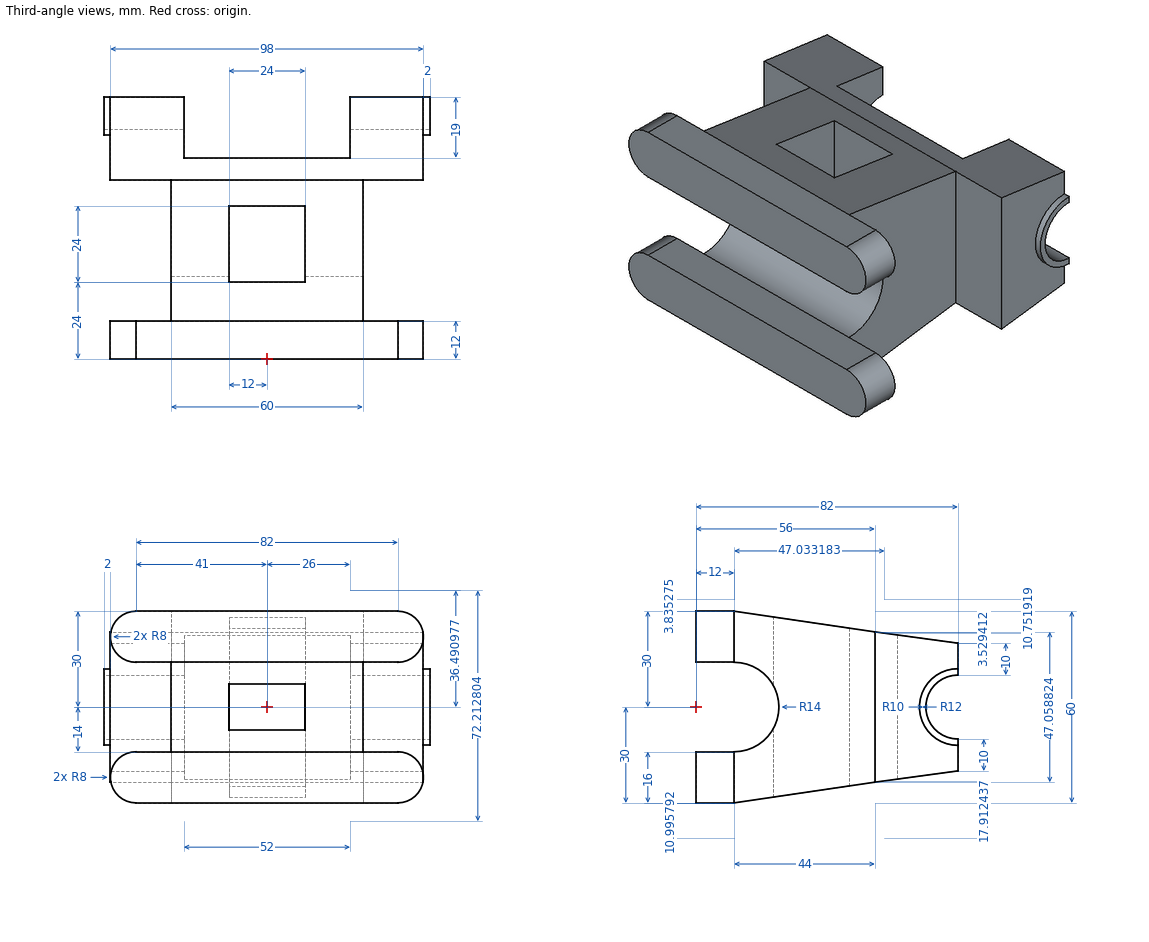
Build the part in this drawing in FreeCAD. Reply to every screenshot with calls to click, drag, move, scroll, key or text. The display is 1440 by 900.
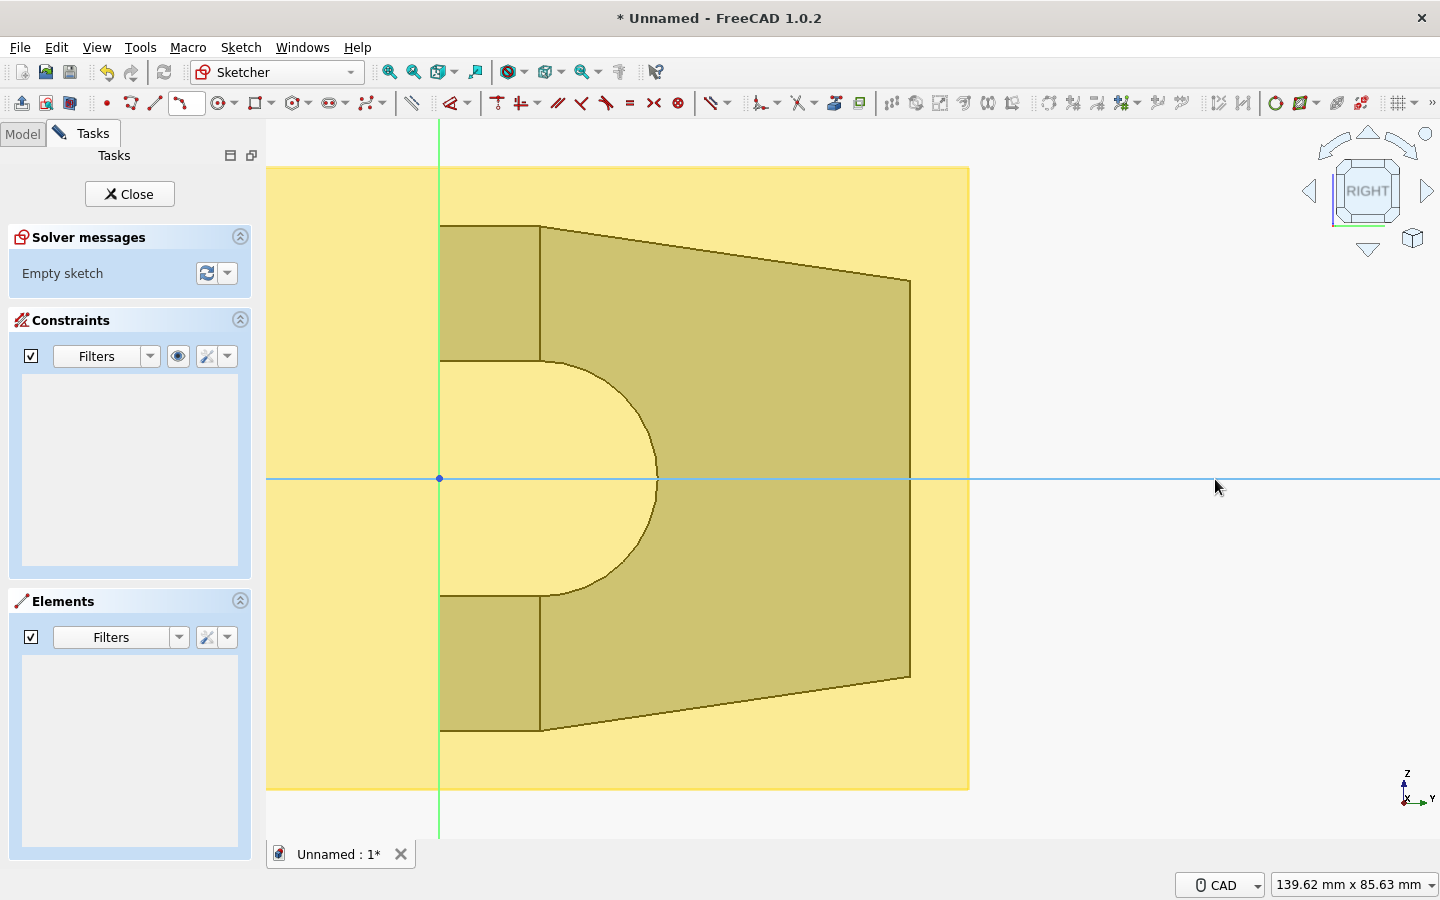
click(132, 104)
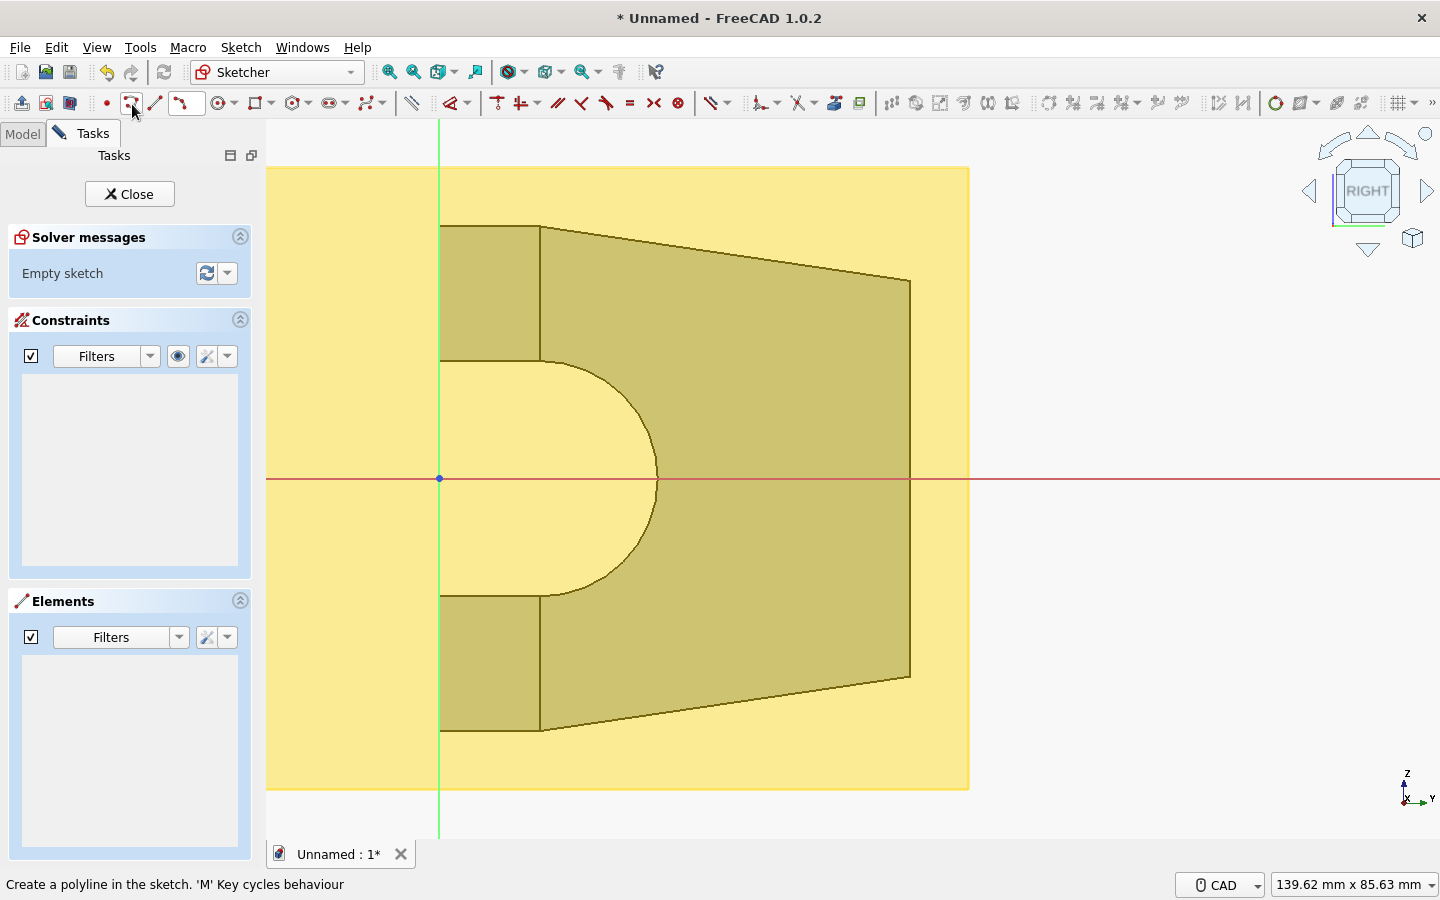
click(1129, 395)
click(1129, 311)
click(910, 281)
click(910, 677)
click(1129, 647)
click(1129, 563)
right_click(1129, 563)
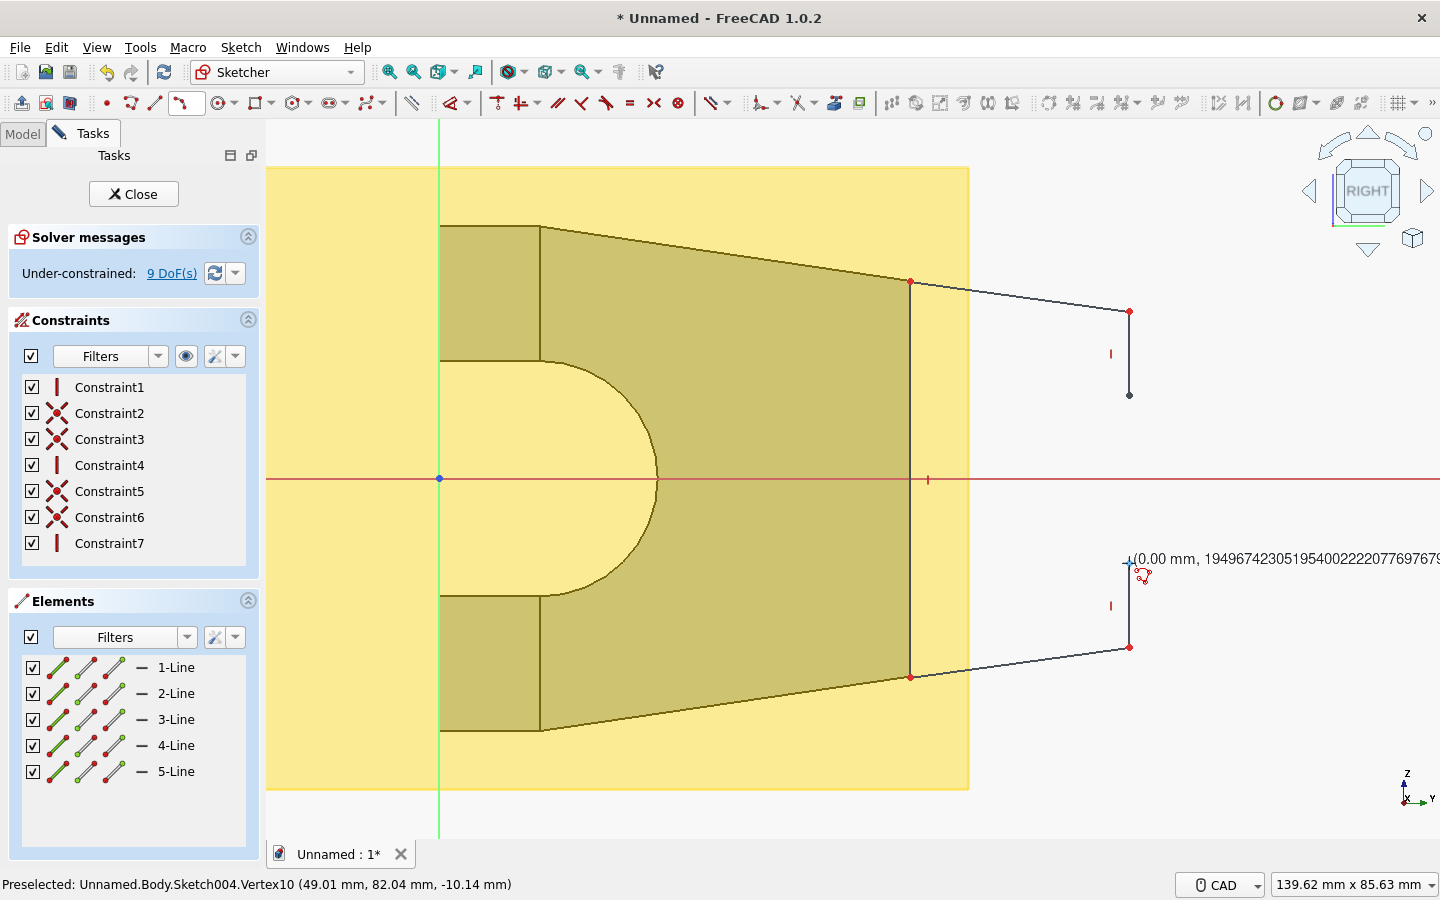
click(180, 104)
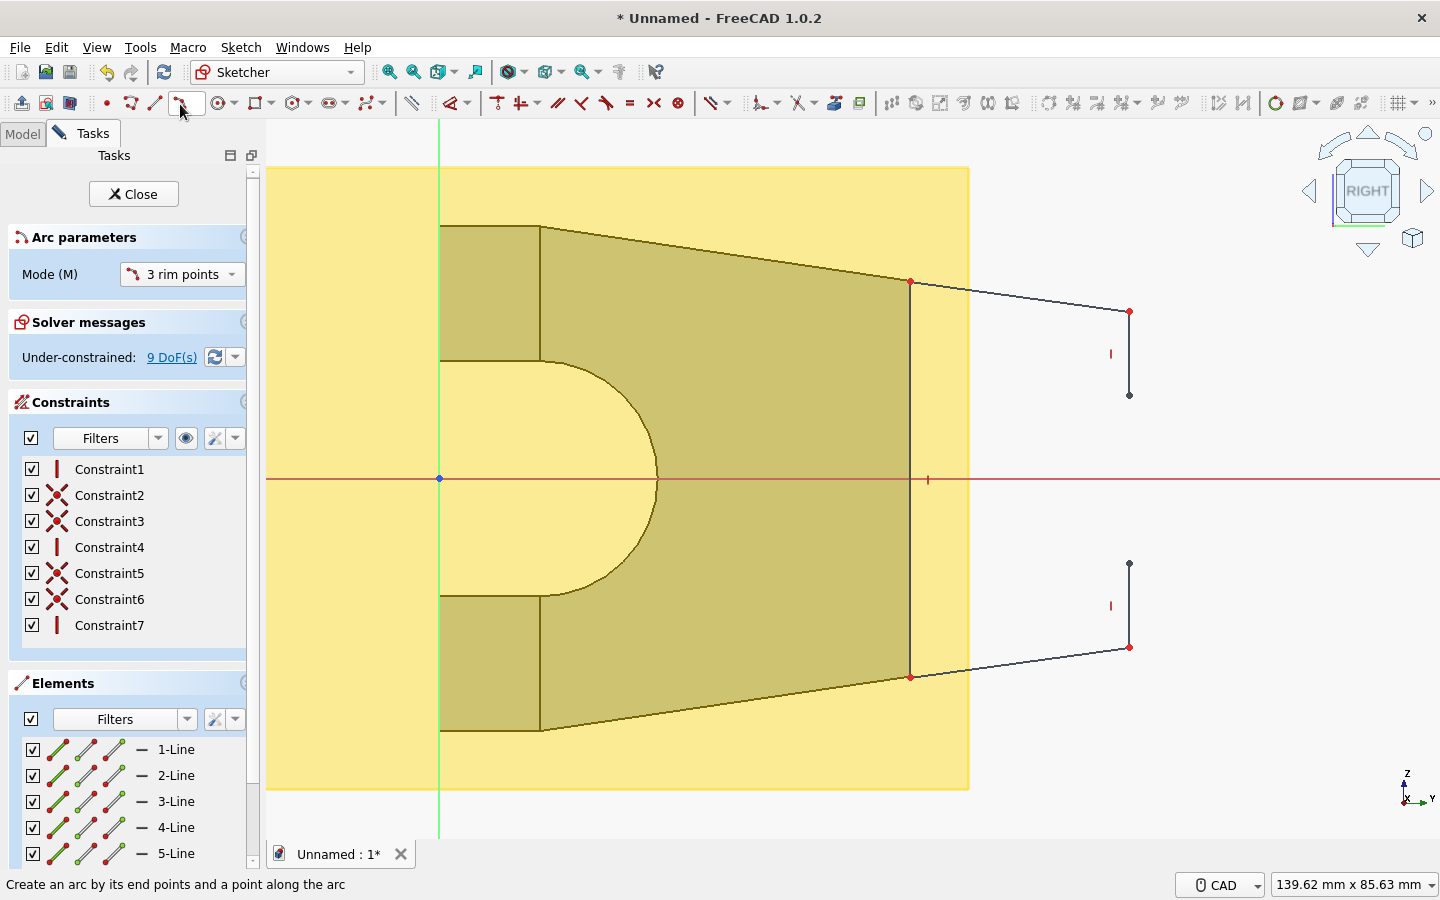
click(1129, 564)
click(1129, 396)
click(1049, 453)
key(Escape)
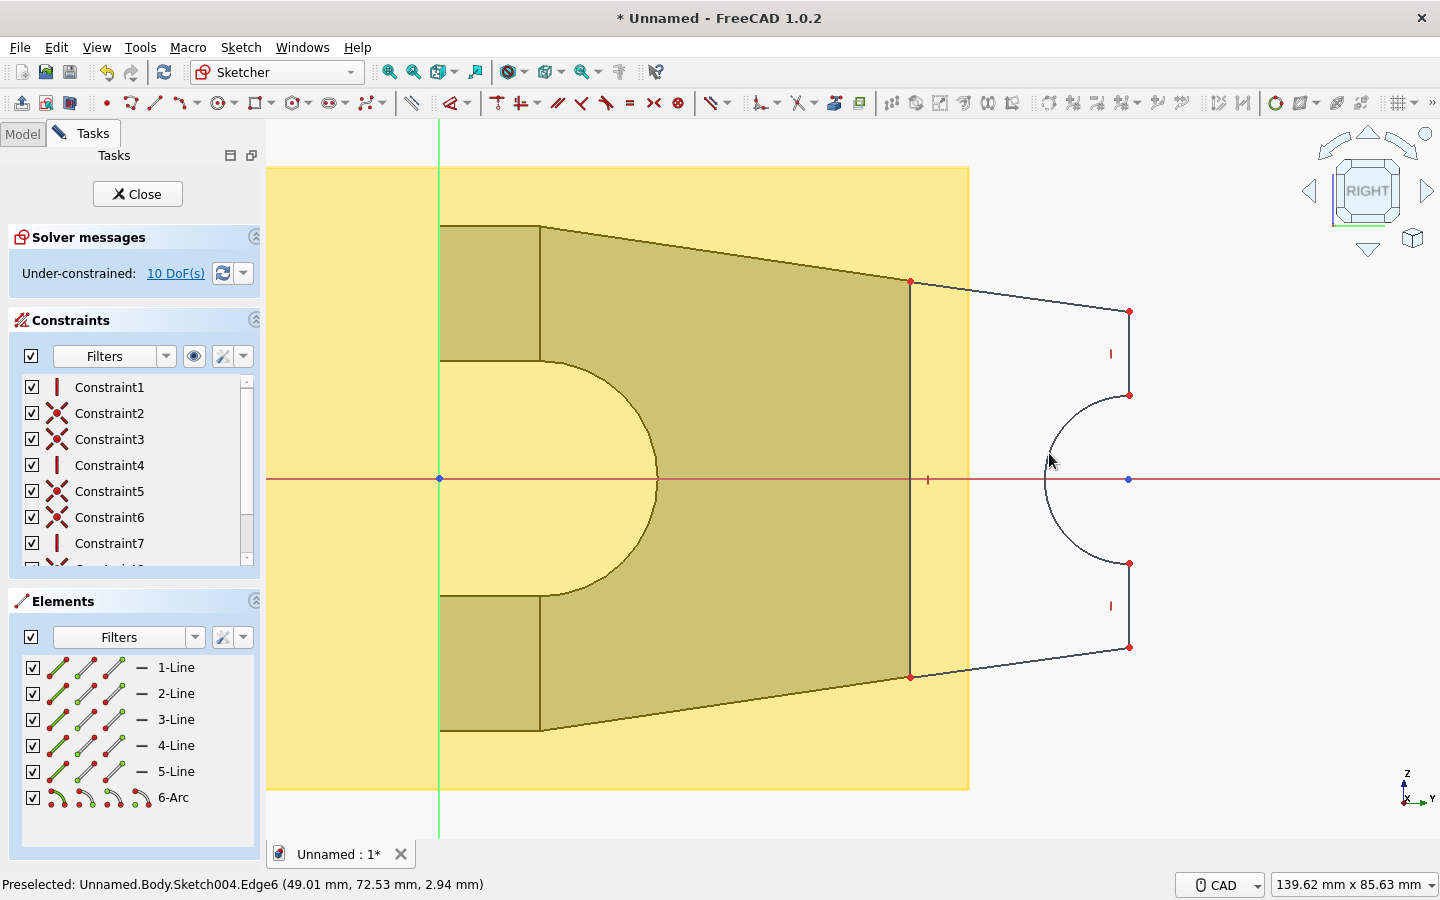
click(1129, 480)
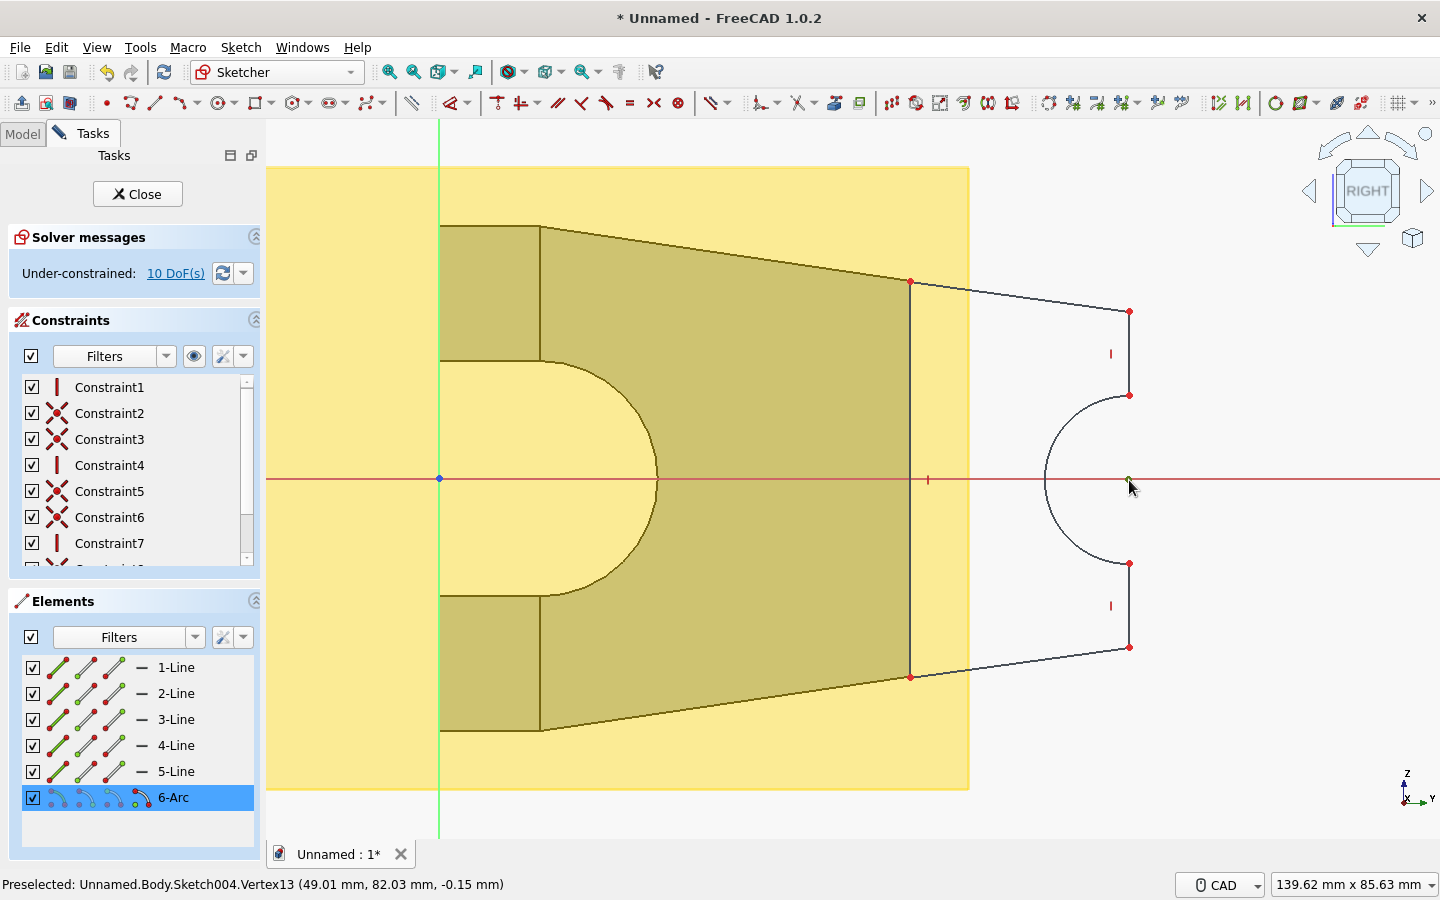
click(364, 479)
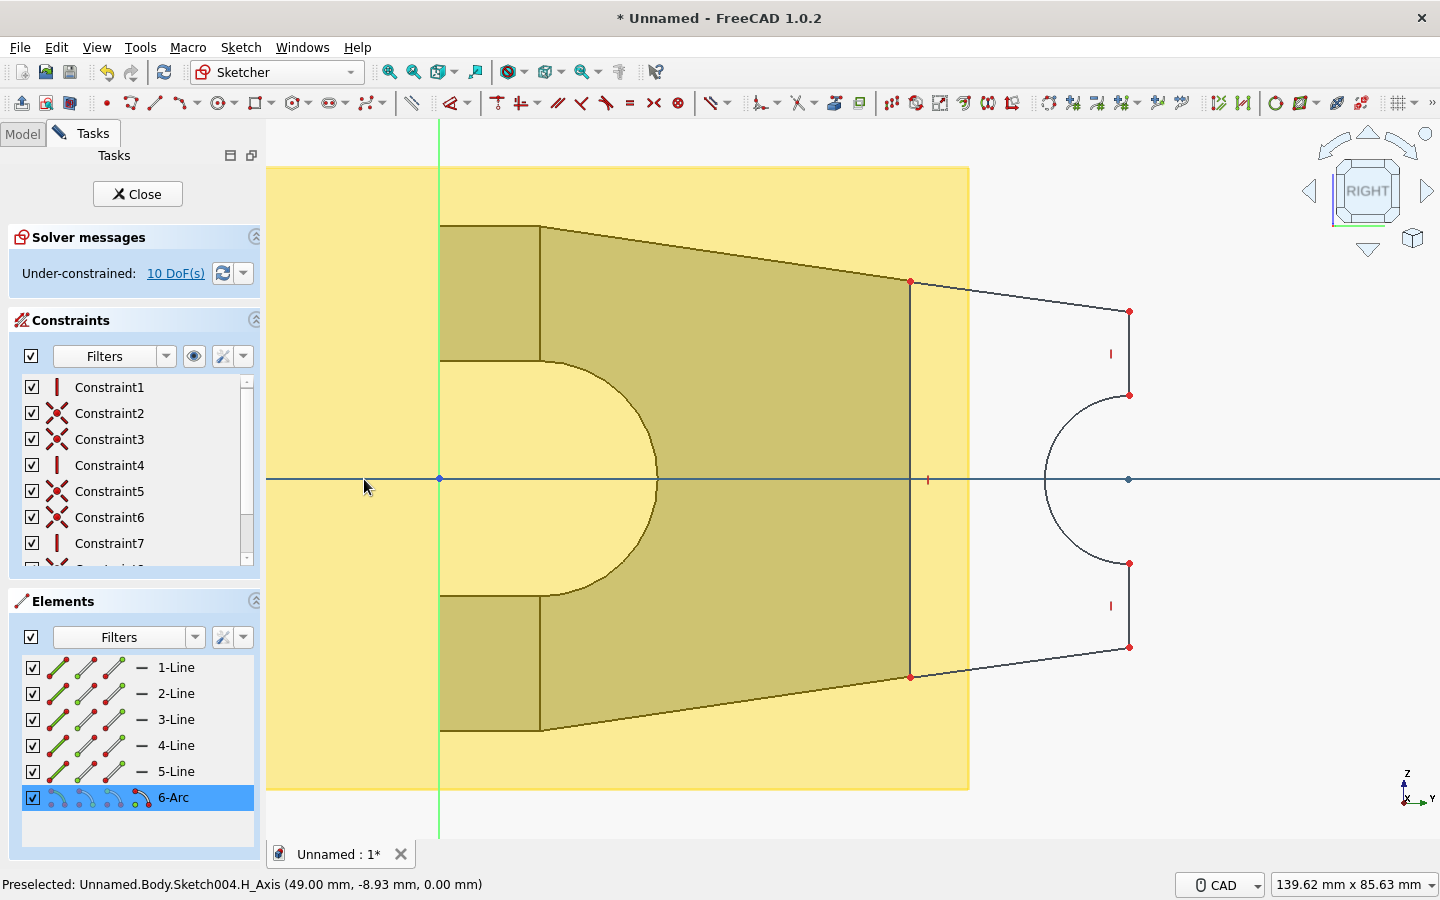
click(498, 104)